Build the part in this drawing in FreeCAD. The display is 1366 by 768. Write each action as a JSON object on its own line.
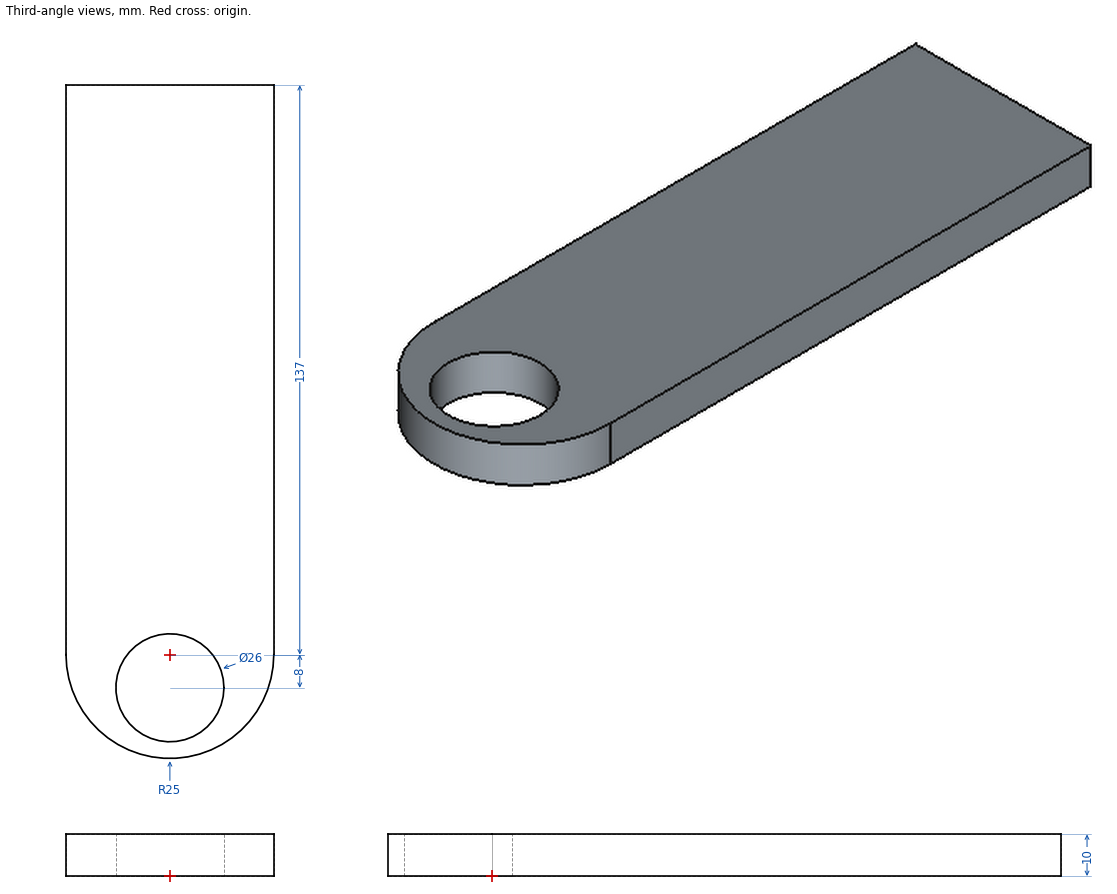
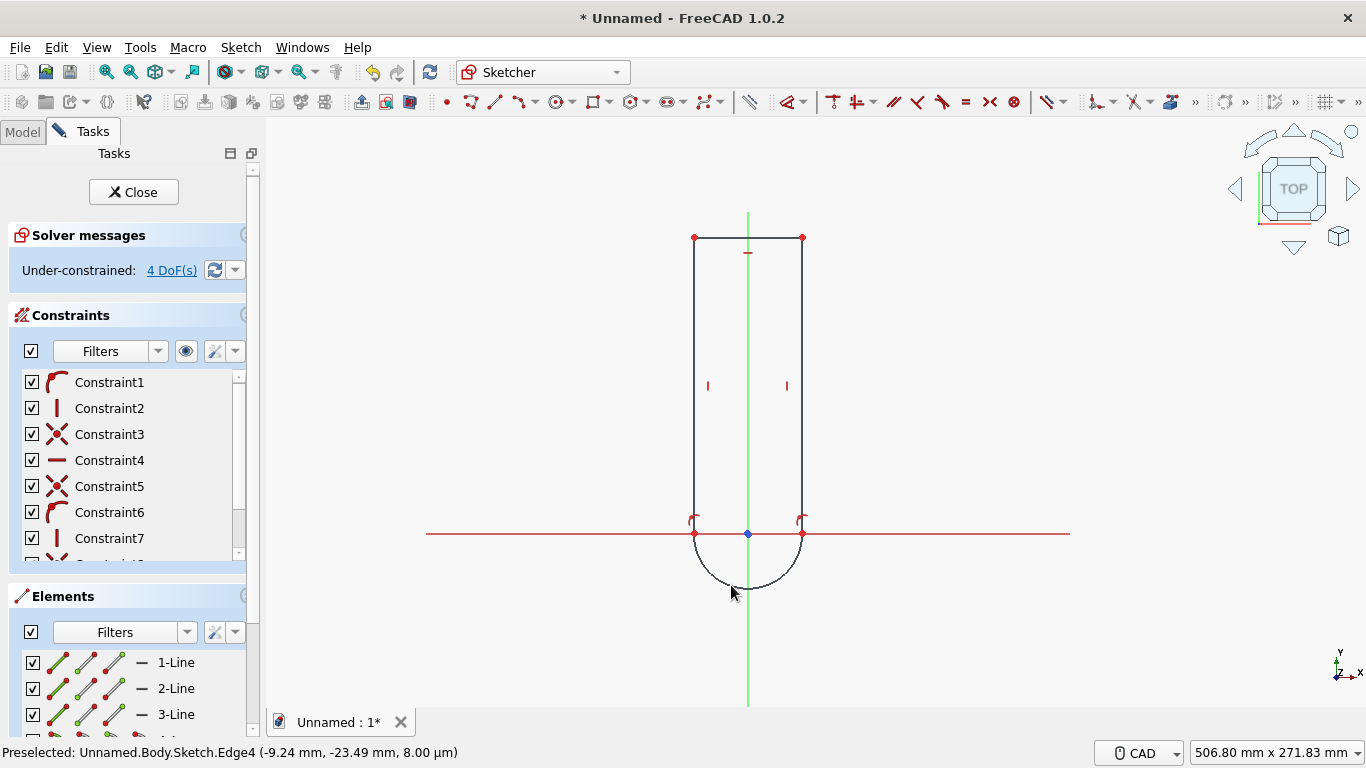
{"action": "left_click", "coordinate": [802, 445]}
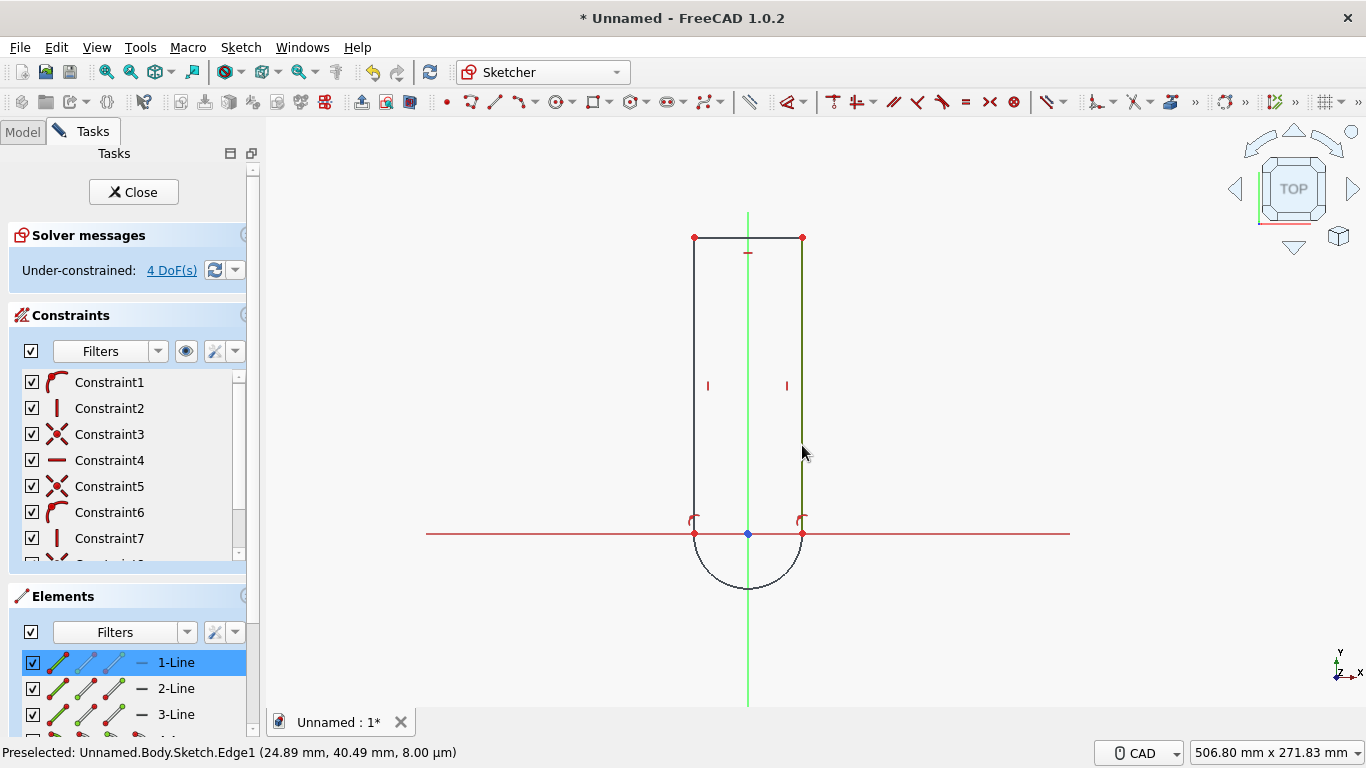
{"action": "left_click", "coordinate": [716, 578]}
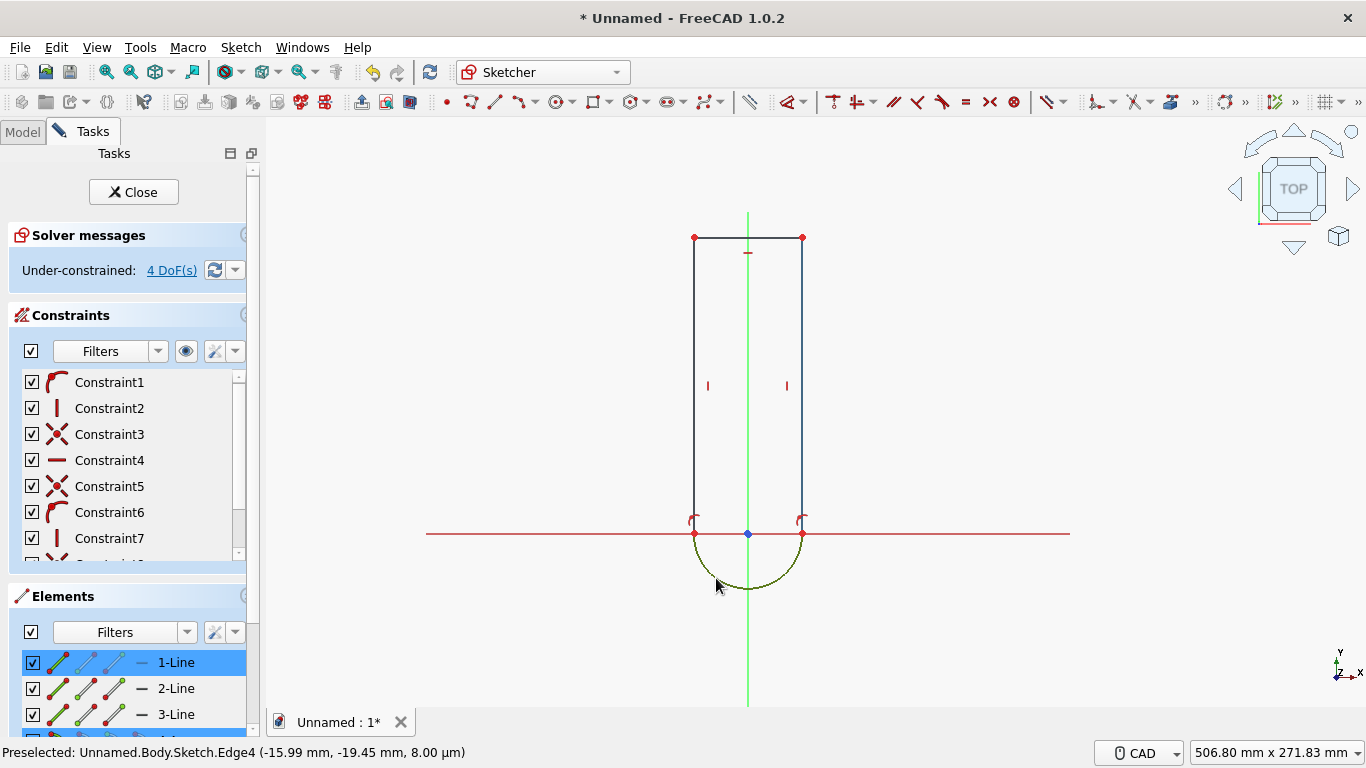
{"action": "left_click", "coordinate": [942, 102]}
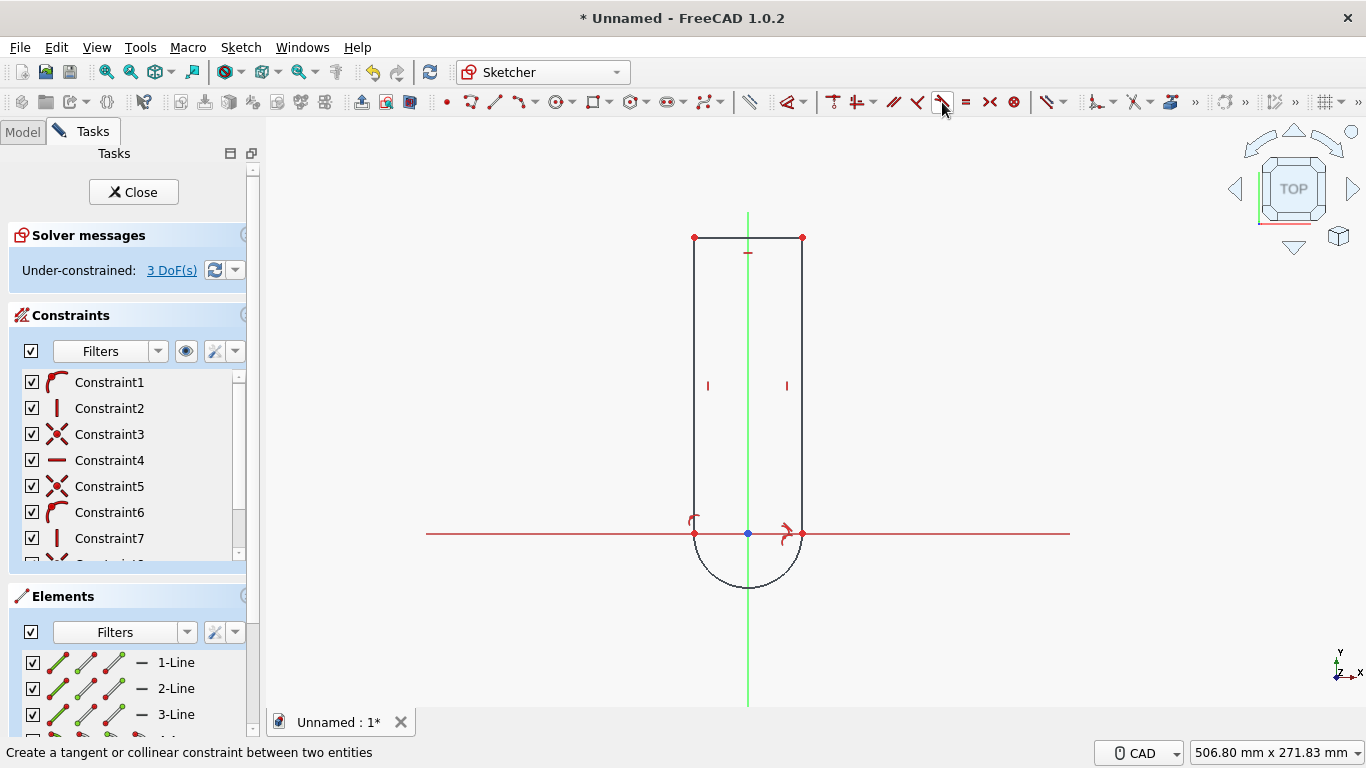
{"action": "left_click", "coordinate": [748, 534]}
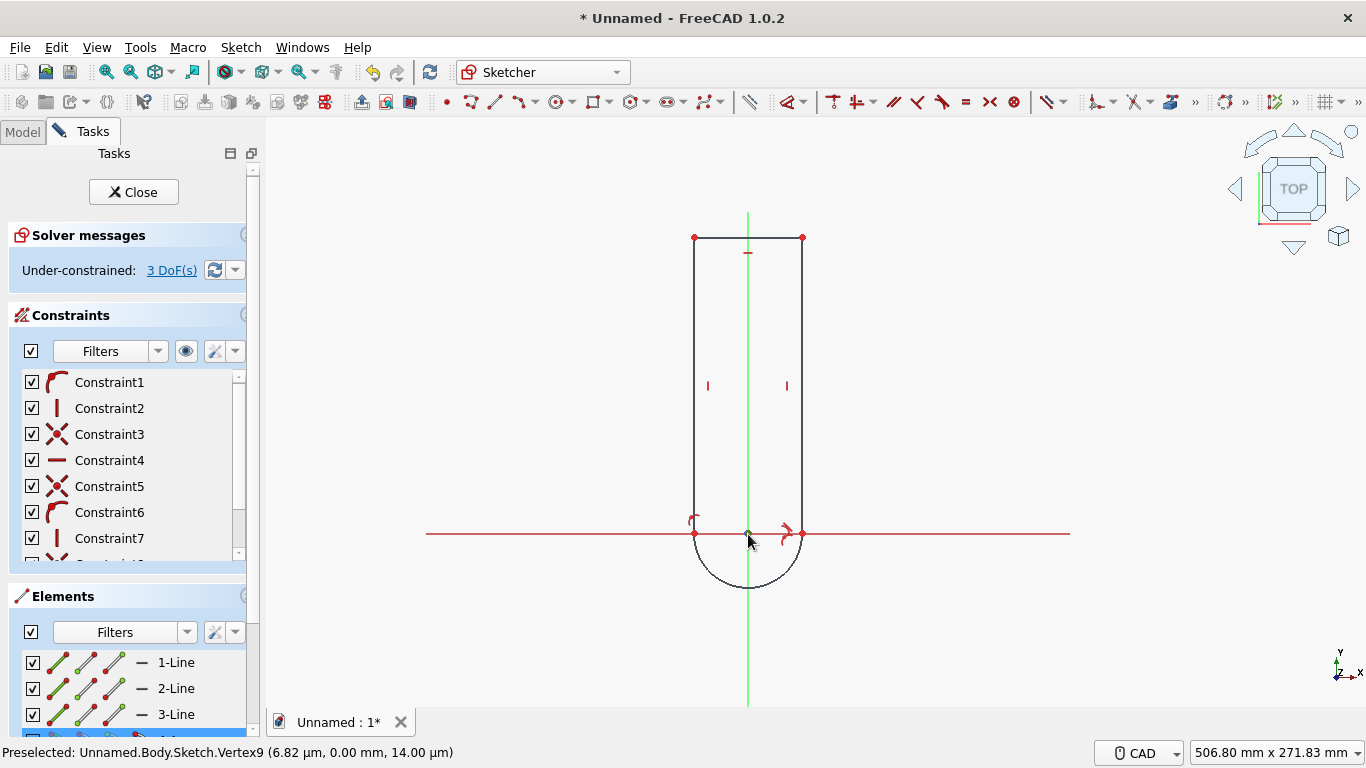
{"action": "left_click", "coordinate": [748, 641]}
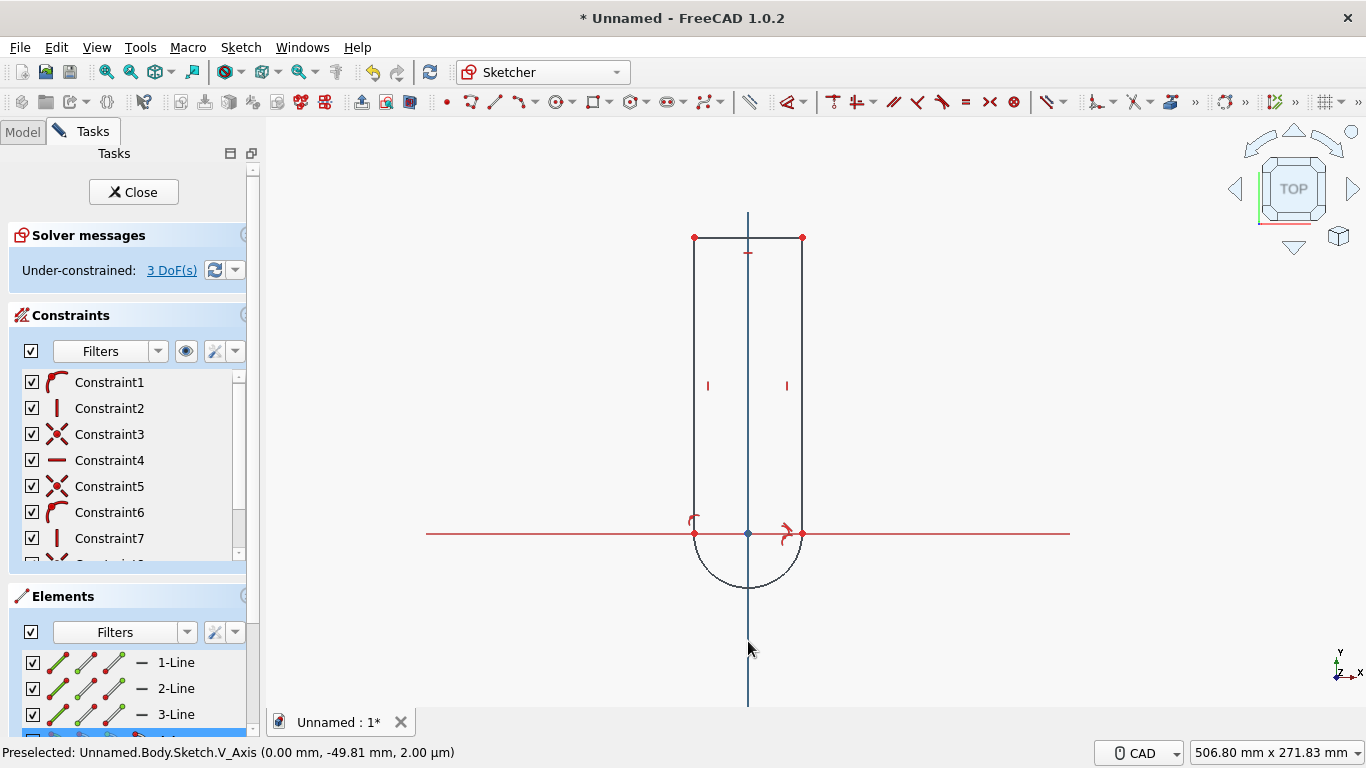
{"action": "left_click", "coordinate": [834, 102]}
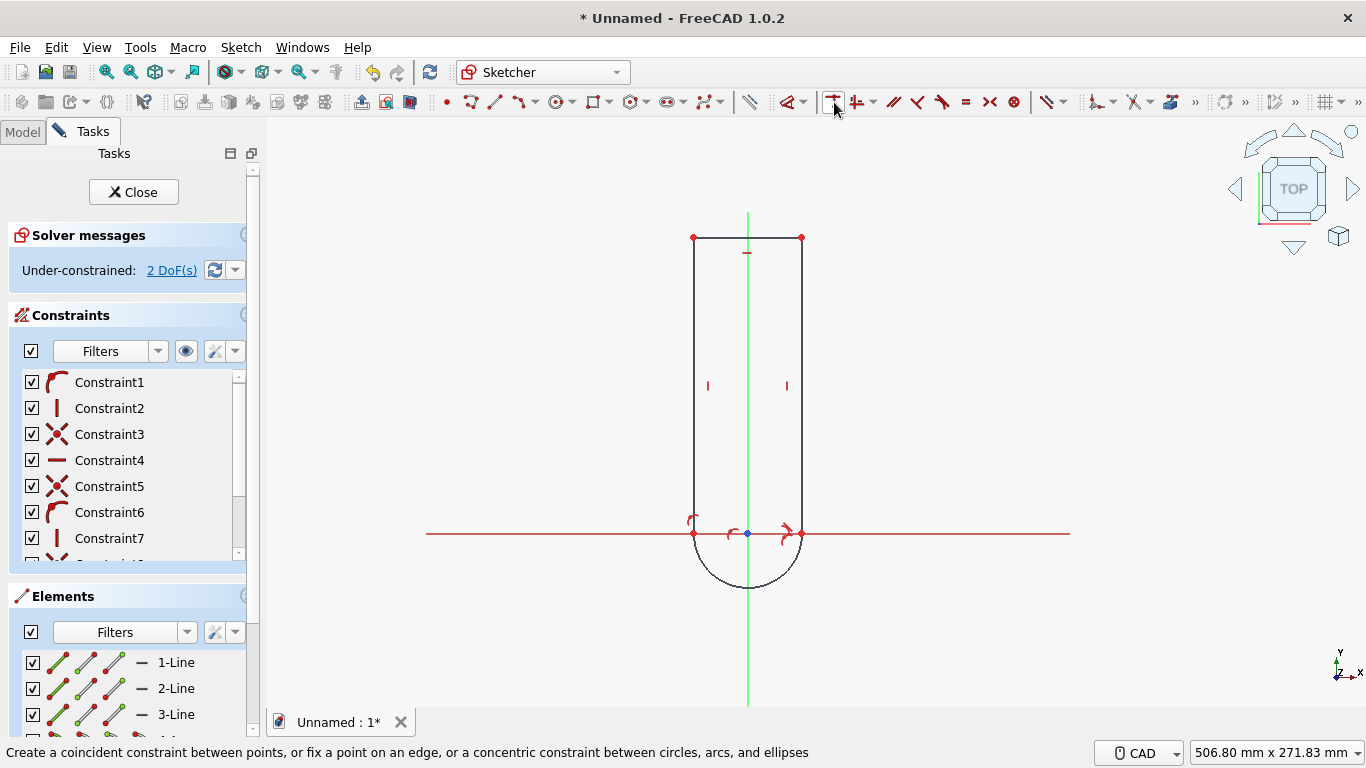
{"action": "left_click", "coordinate": [716, 578]}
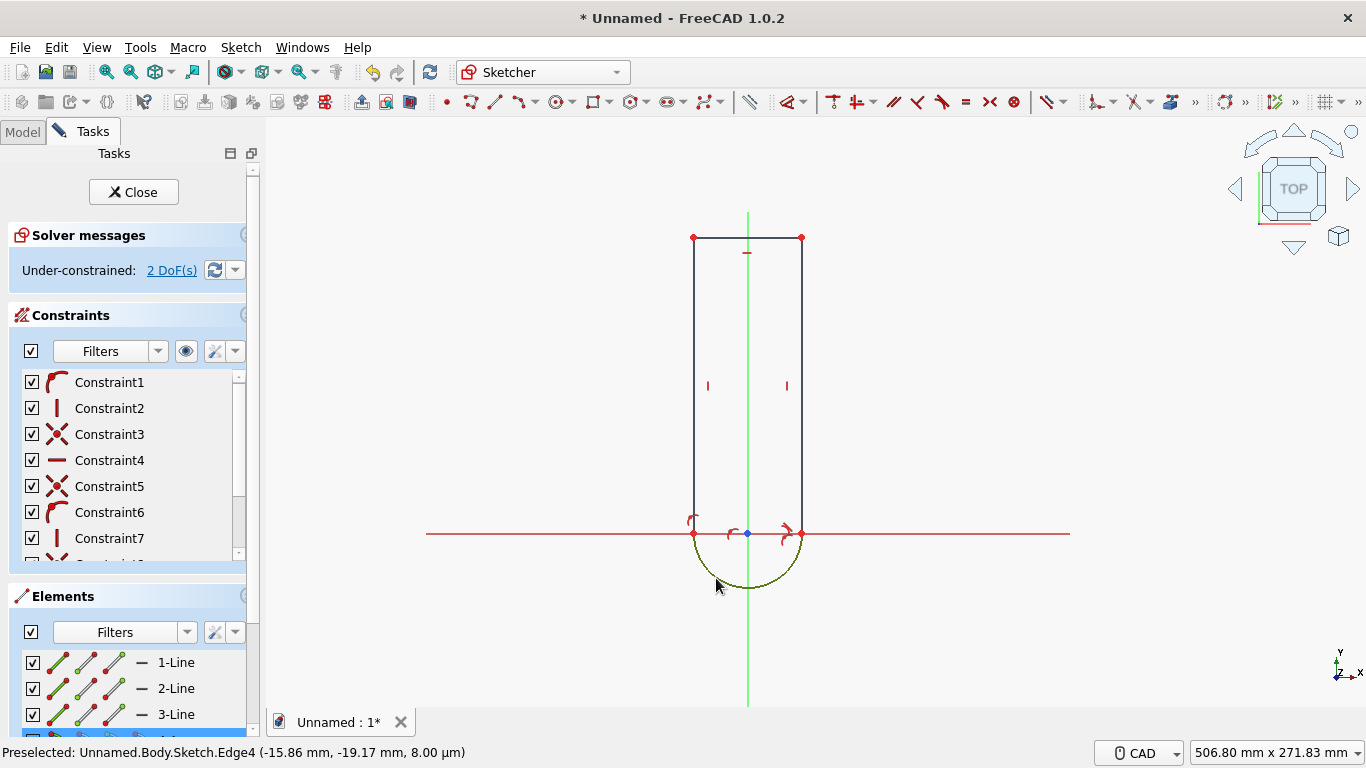
{"action": "key", "text": "k r"}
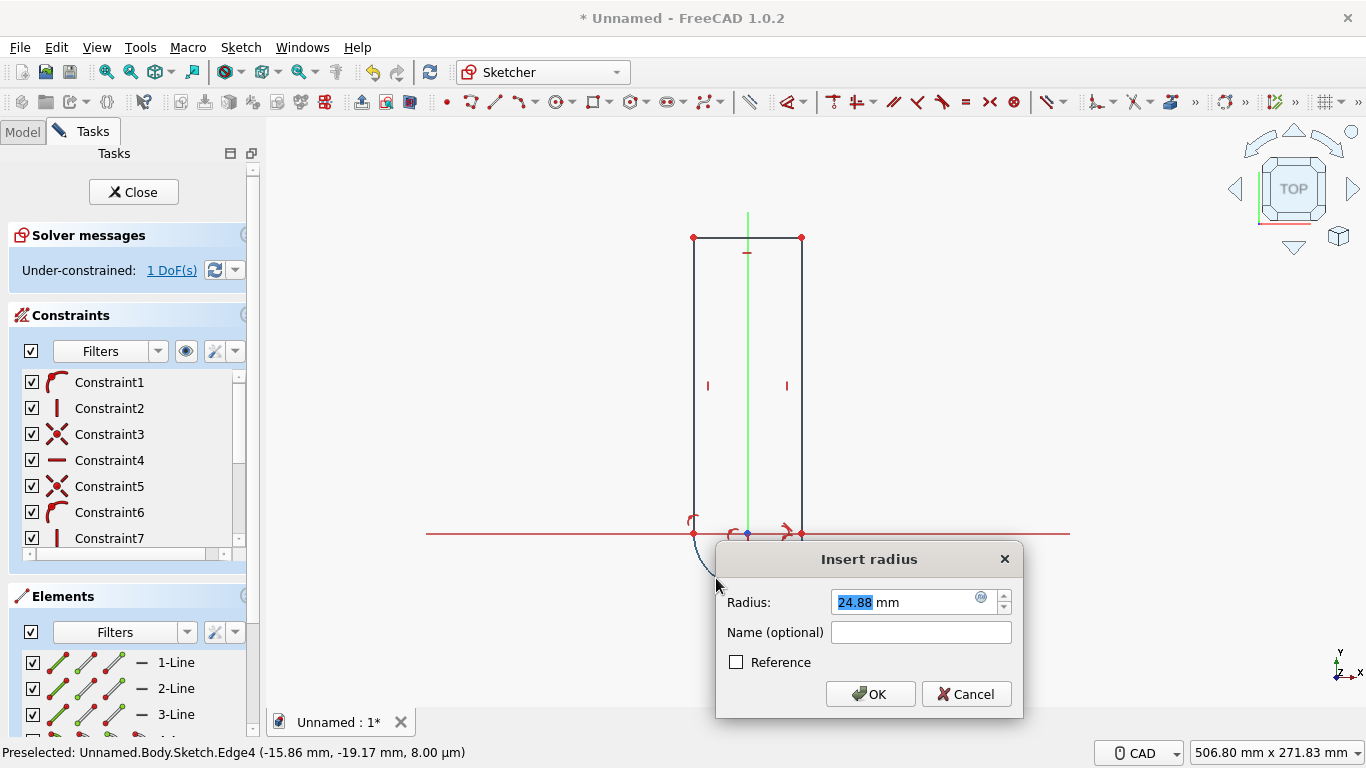
{"action": "type", "text": "25"}
{"action": "key", "text": "Return"}